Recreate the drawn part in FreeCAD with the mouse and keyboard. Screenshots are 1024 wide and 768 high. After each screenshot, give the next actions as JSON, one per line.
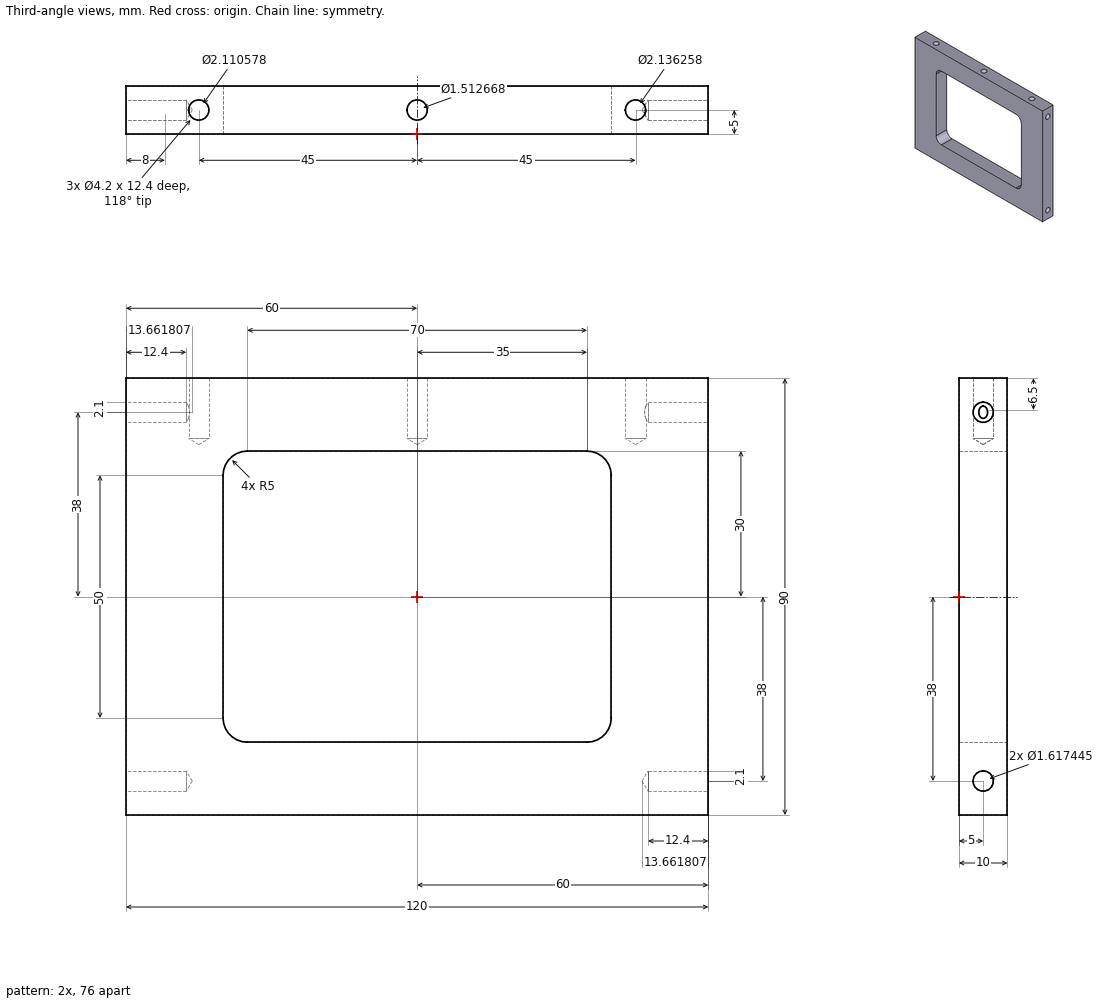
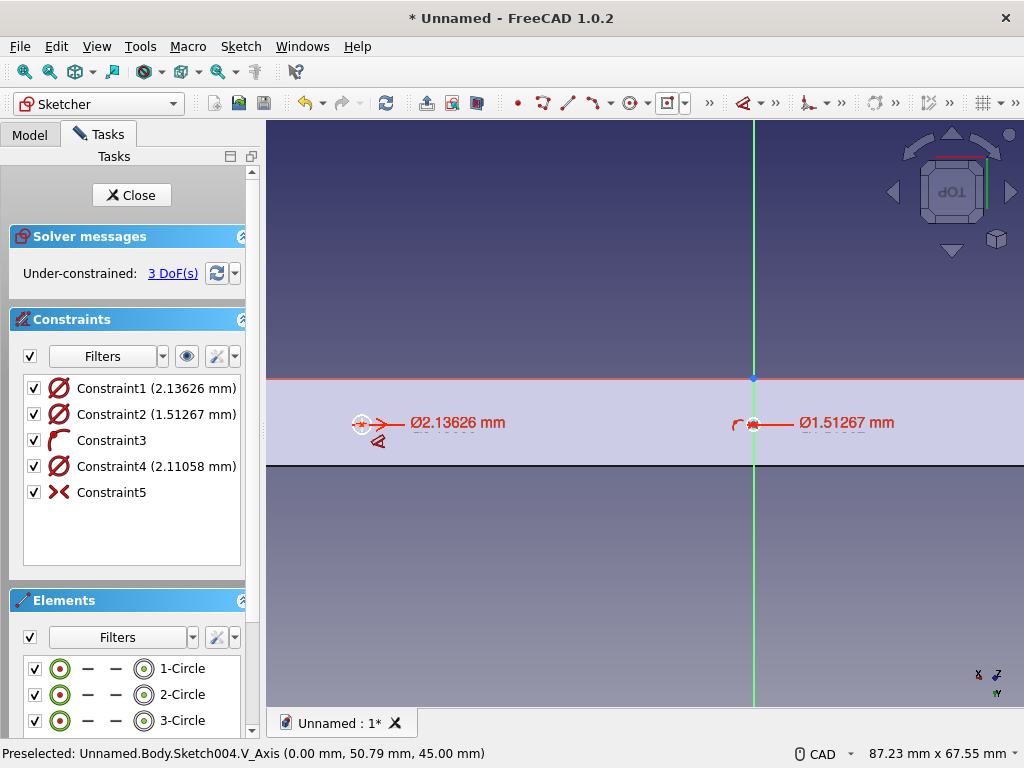
{"action": "left_click", "coordinate": [362, 425]}
{"action": "left_click", "coordinate": [328, 402]}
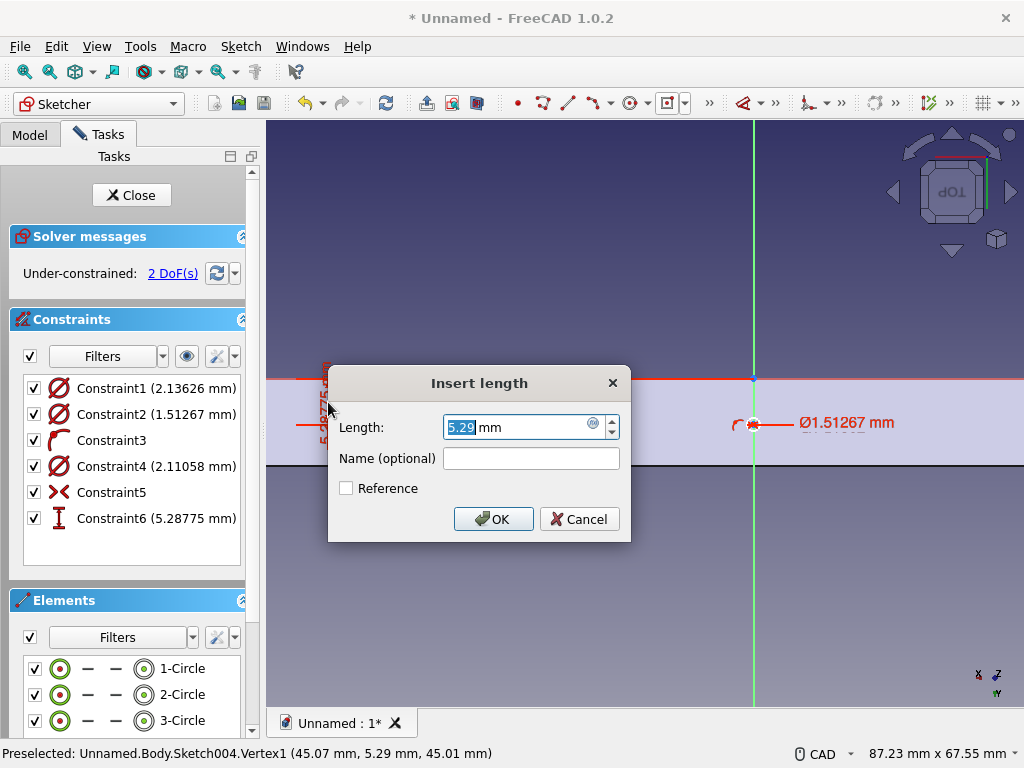
{"action": "type", "text": "5"}
{"action": "key", "text": "Return"}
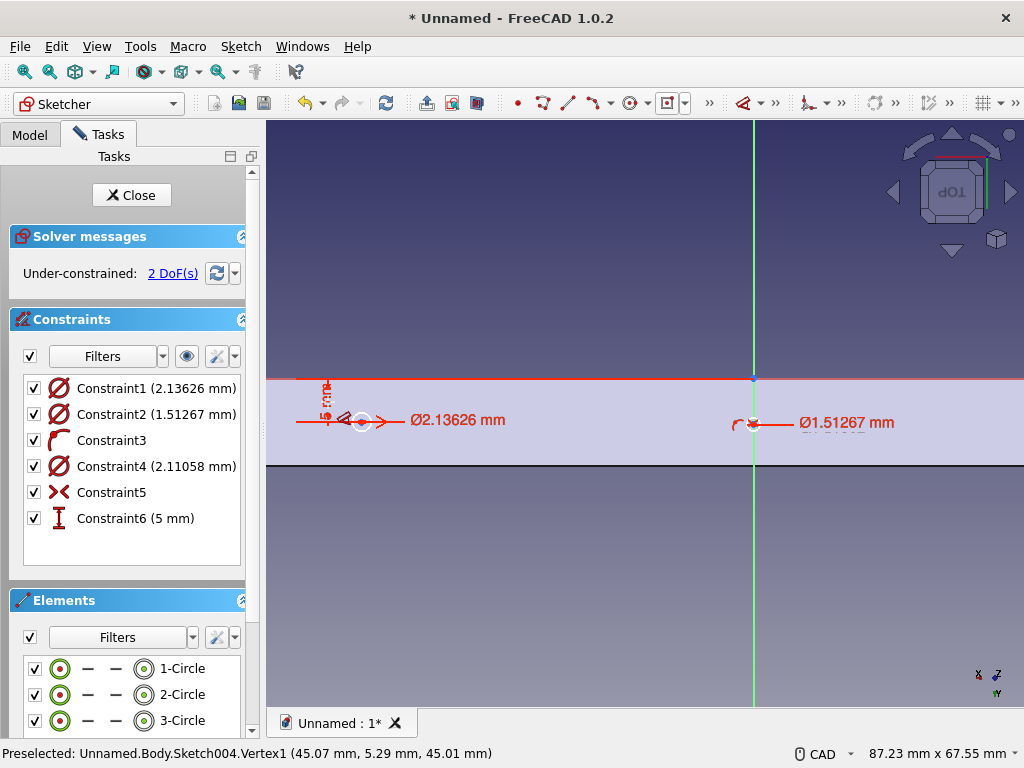
{"action": "left_click", "coordinate": [754, 425]}
{"action": "left_click", "coordinate": [788, 402]}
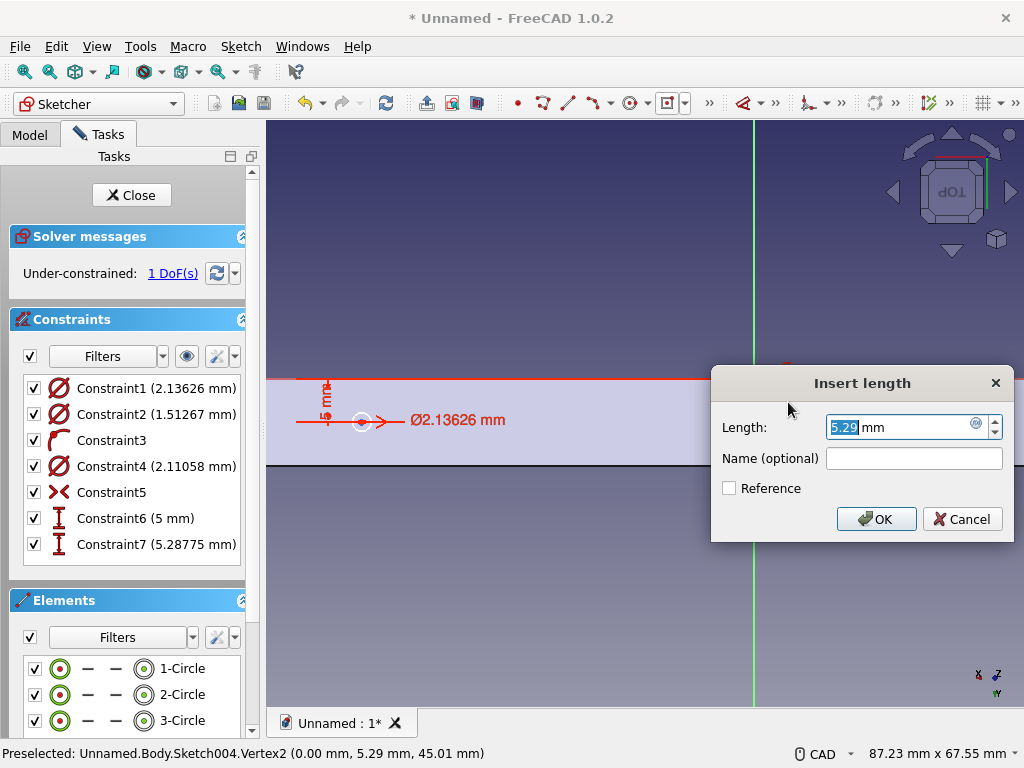
{"action": "type", "text": "5"}
{"action": "key", "text": "Return"}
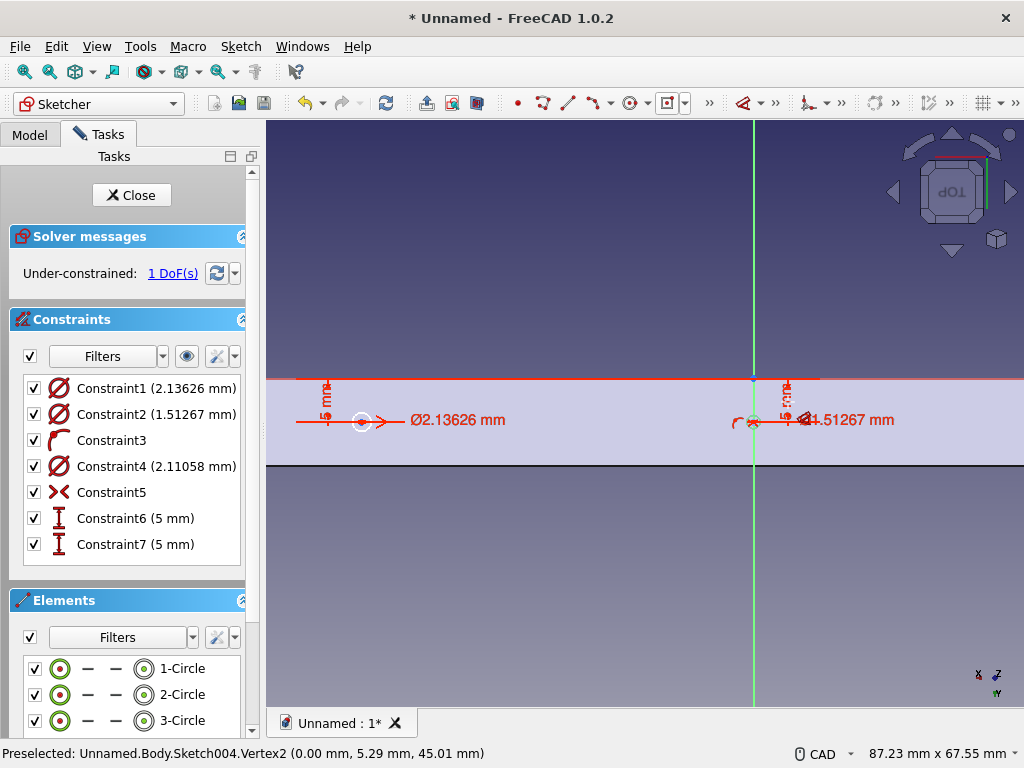
{"action": "left_click", "coordinate": [362, 422]}
{"action": "left_click", "coordinate": [558, 345]}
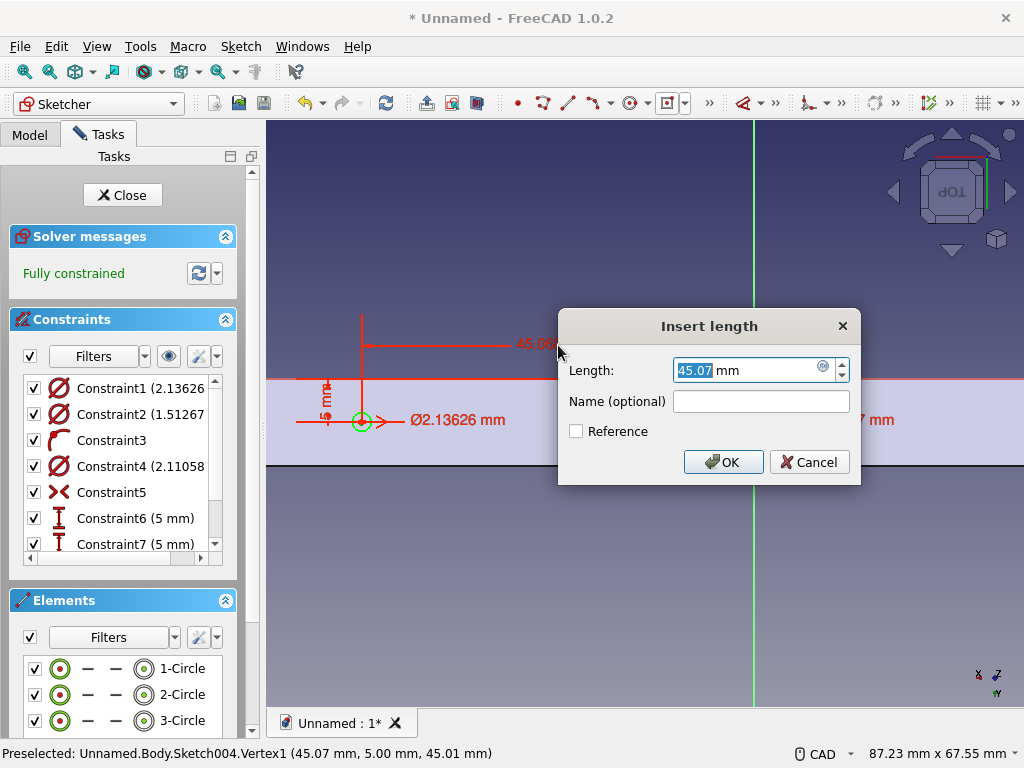
{"action": "type", "text": "45"}
{"action": "key", "text": "Return"}
{"action": "key", "text": "Escape"}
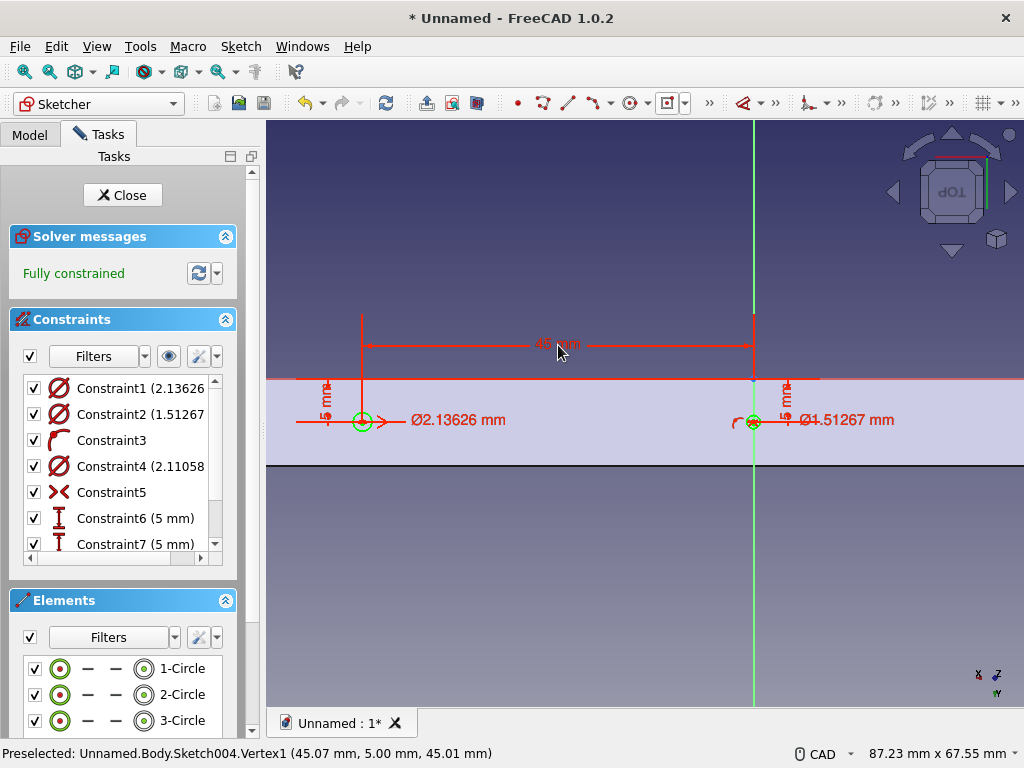
{"action": "left_click", "coordinate": [123, 195]}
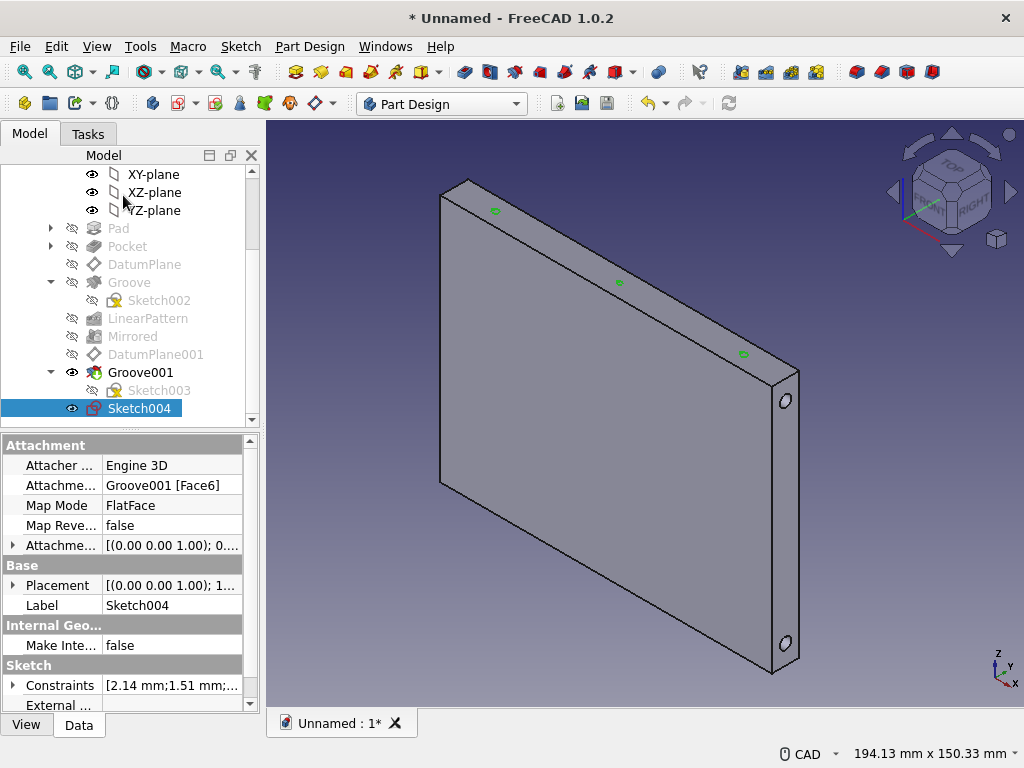
{"action": "left_click", "coordinate": [465, 72]}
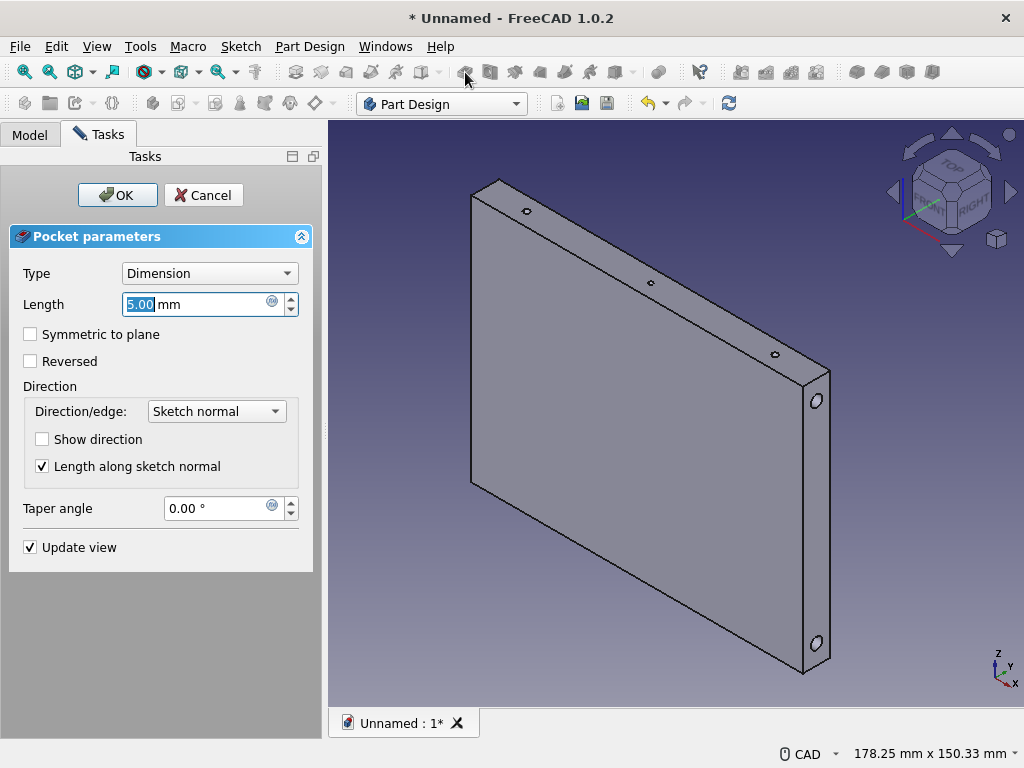
{"action": "type", "text": "6.5"}
{"action": "key", "text": "Tab"}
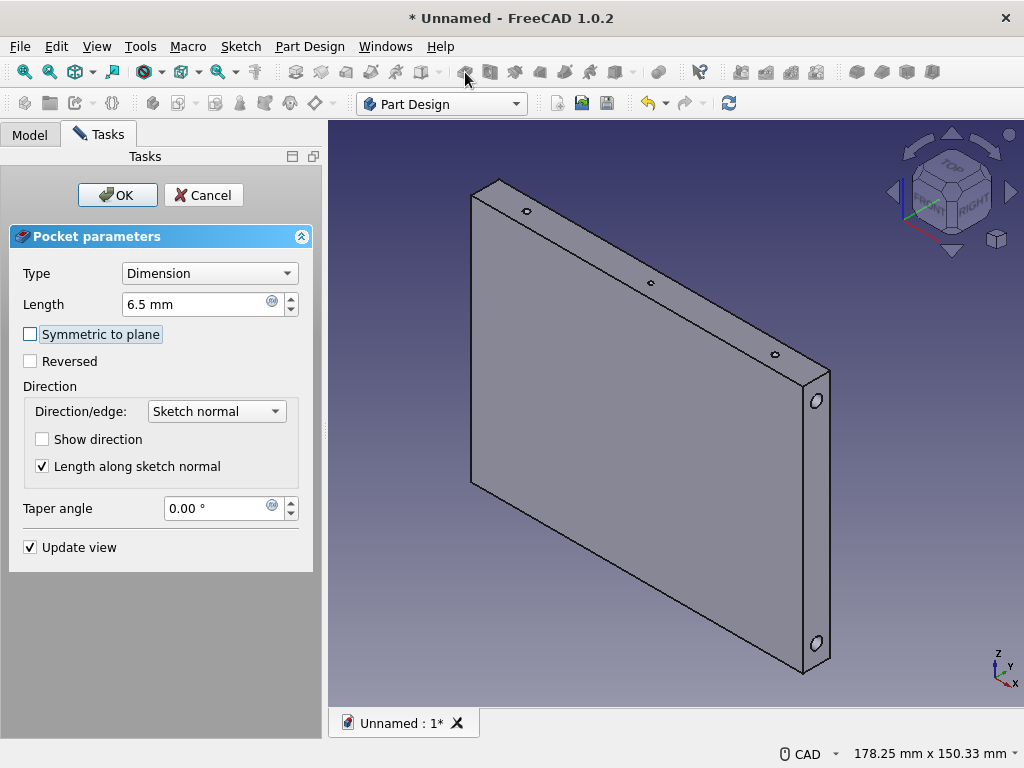
{"action": "left_click", "coordinate": [118, 195]}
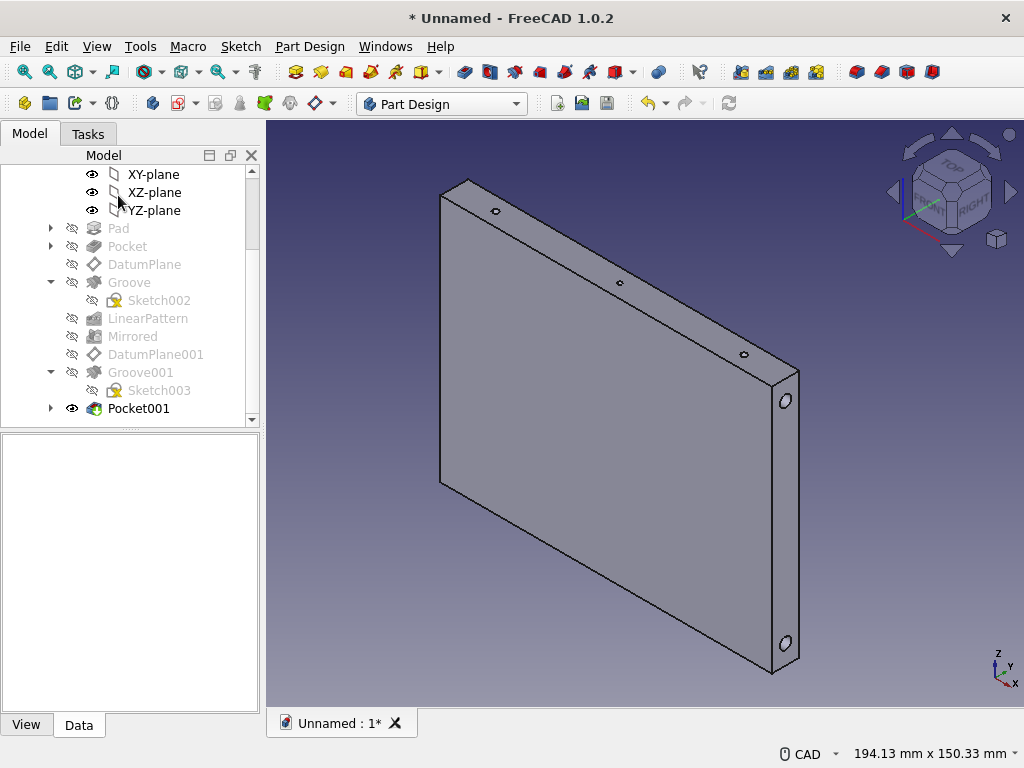
{"action": "left_click", "coordinate": [762, 364]}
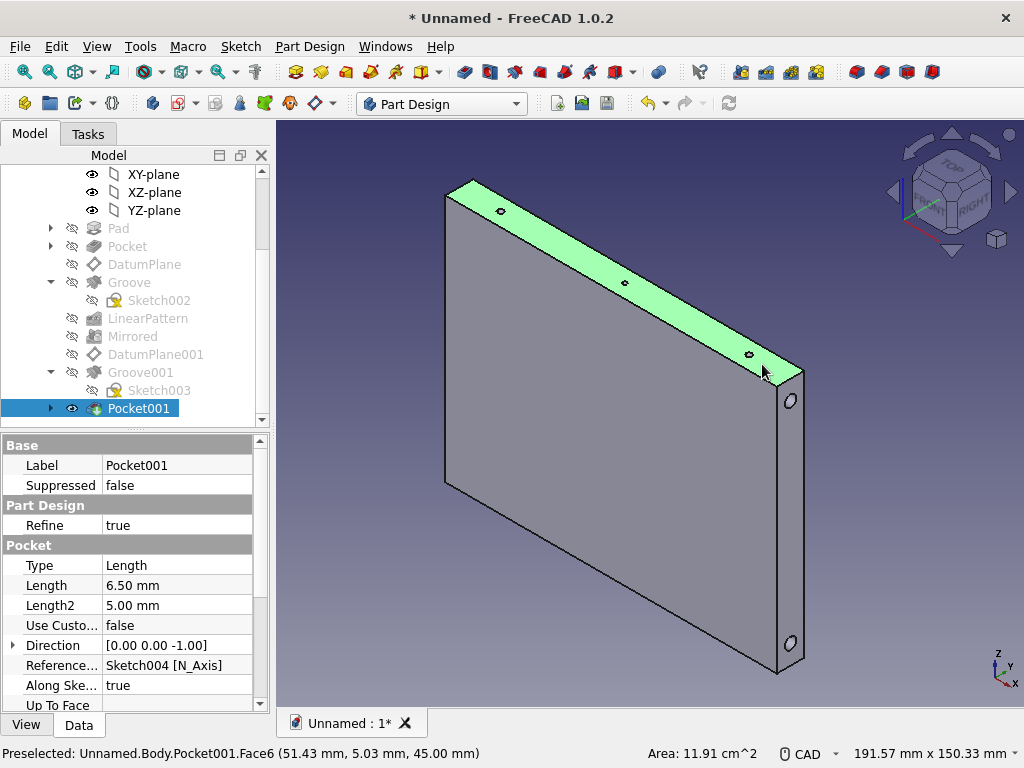
{"action": "left_click", "coordinate": [178, 104]}